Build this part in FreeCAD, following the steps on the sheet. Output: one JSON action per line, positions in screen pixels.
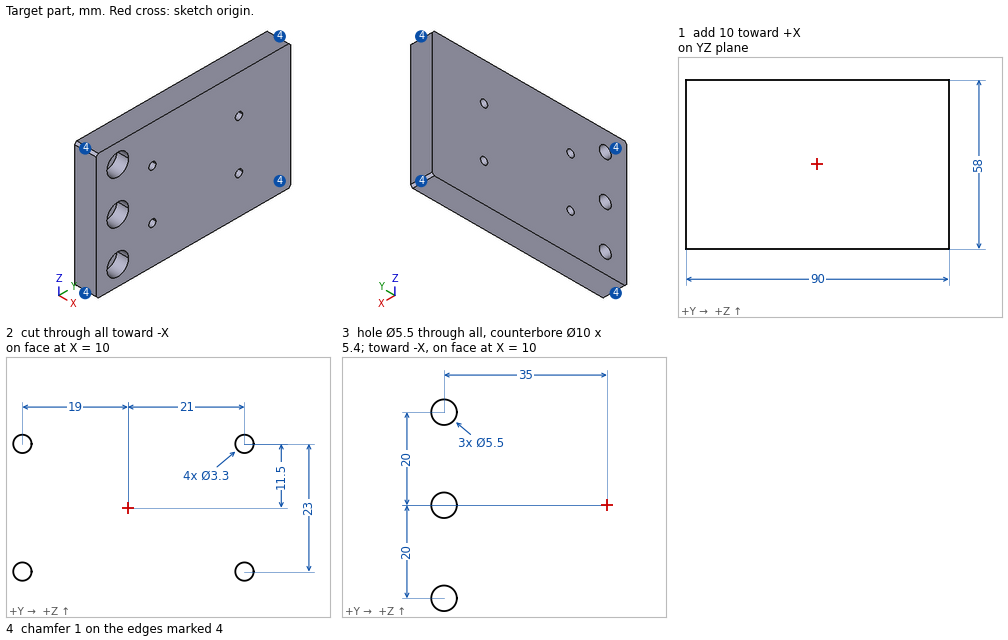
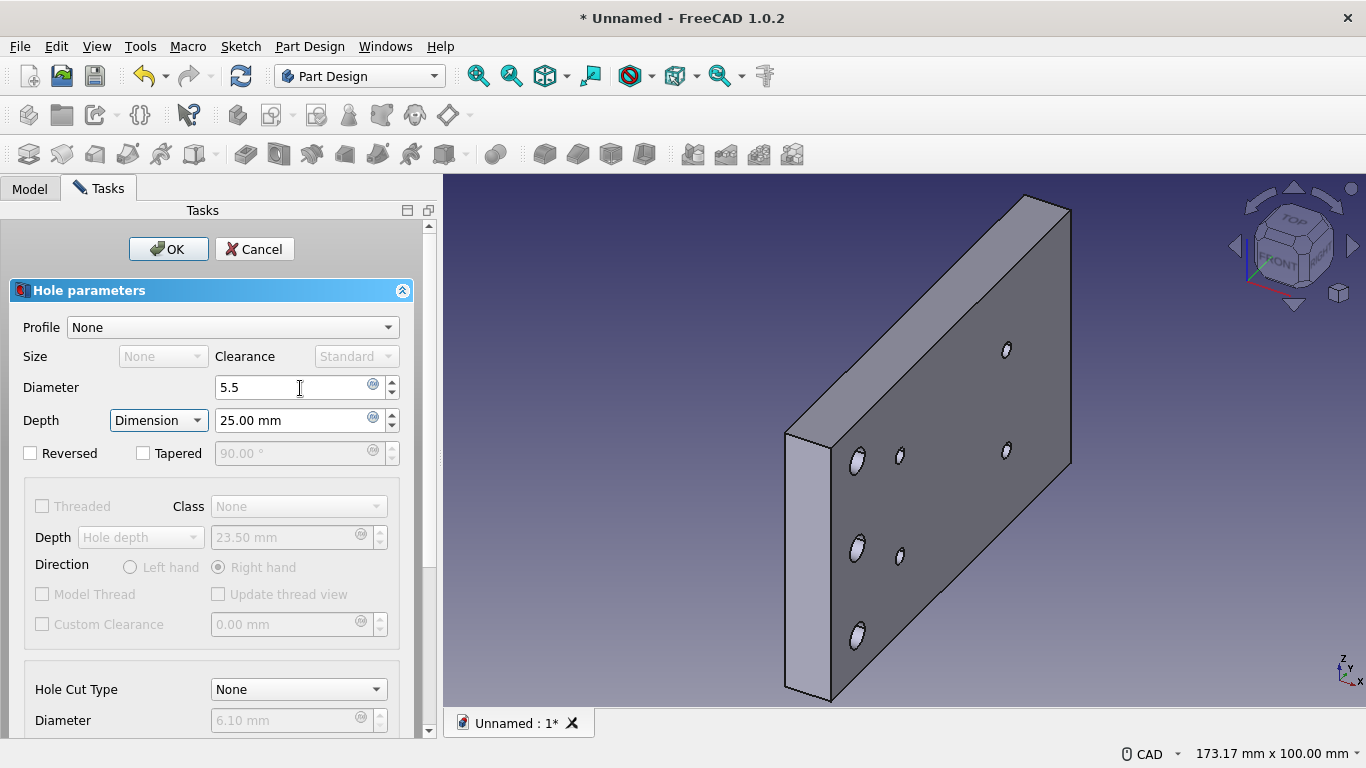
{"action": "left_click", "coordinate": [160, 420]}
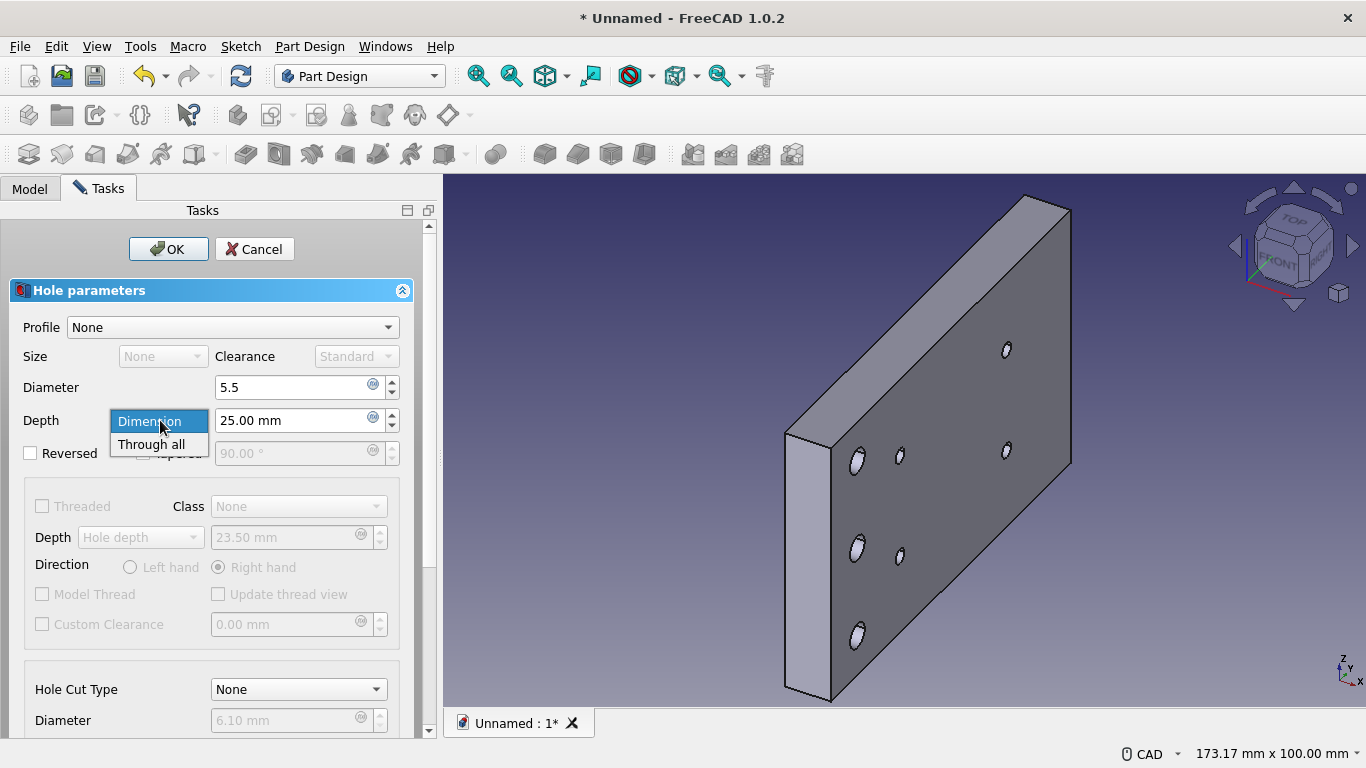
{"action": "left_click", "coordinate": [158, 444]}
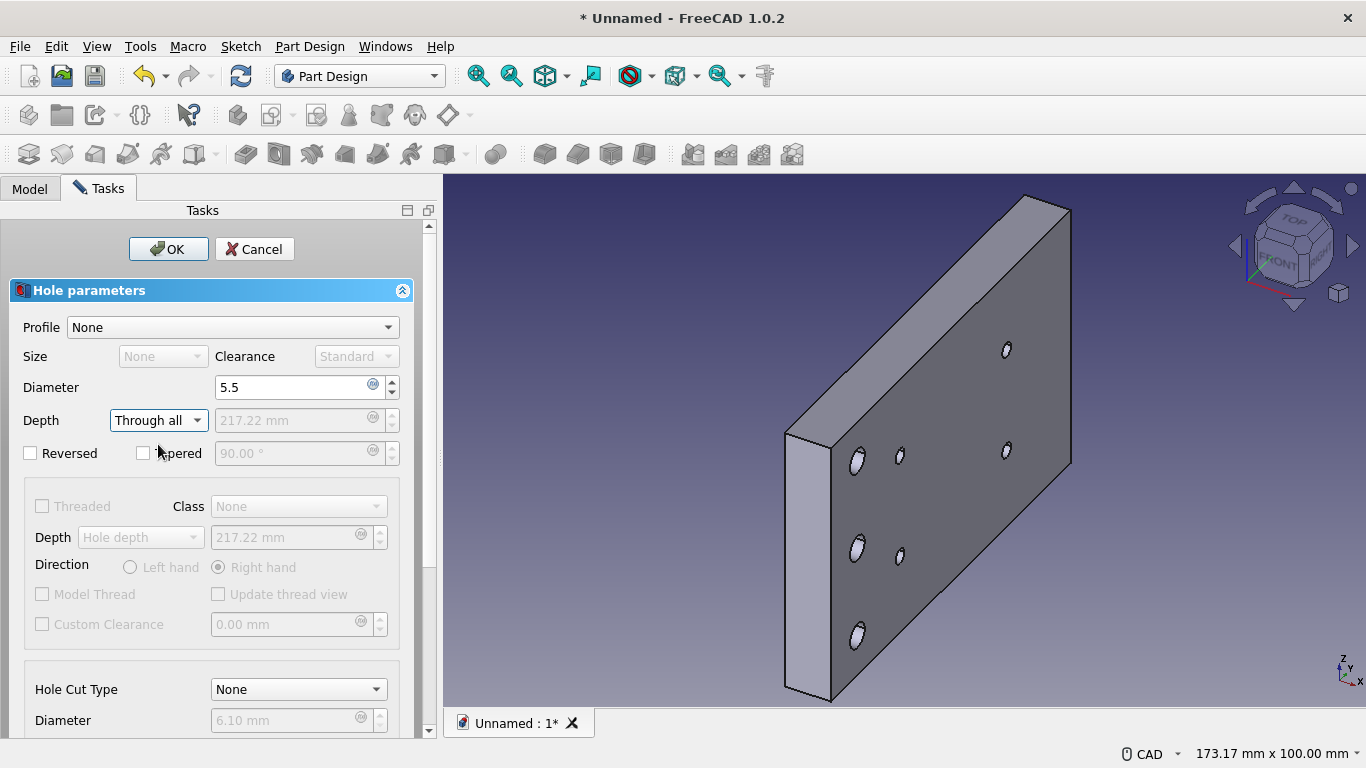
{"action": "left_click", "coordinate": [300, 690]}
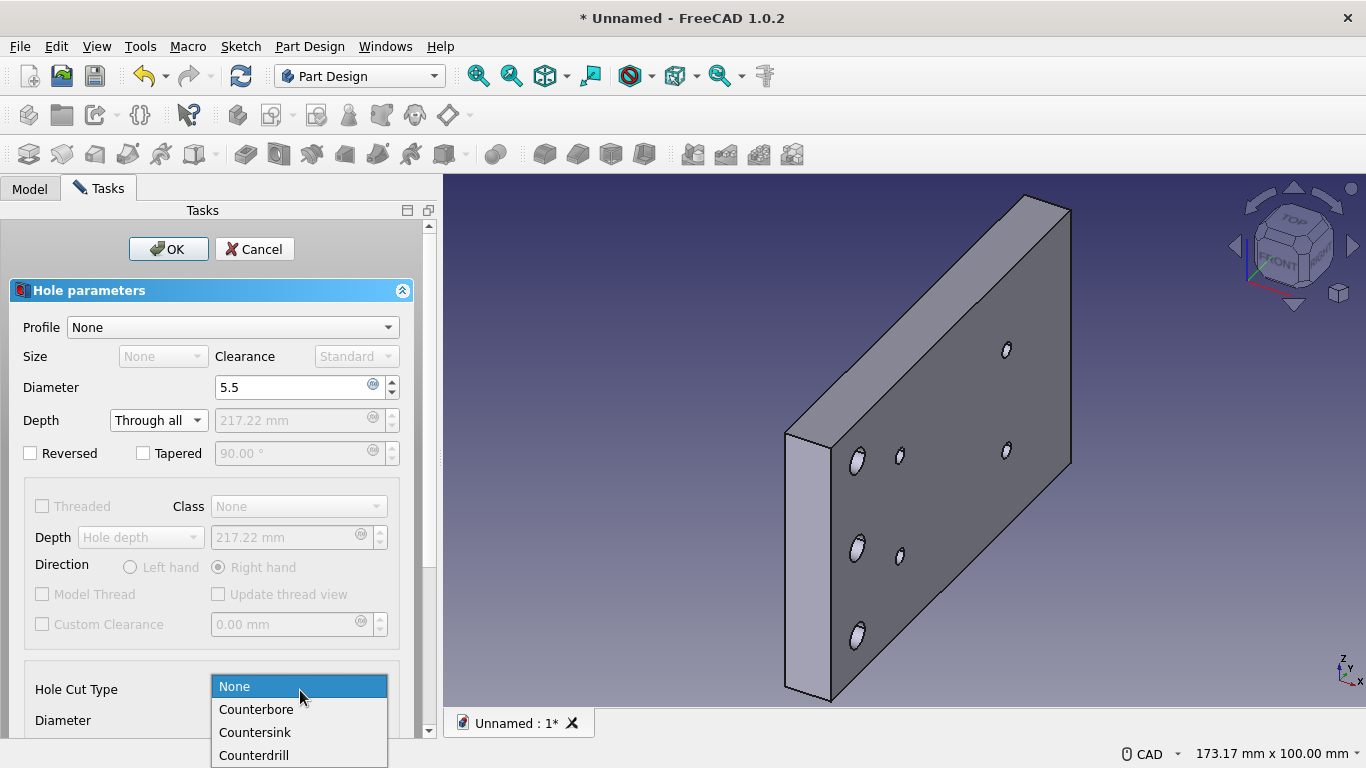
{"action": "left_click", "coordinate": [298, 710]}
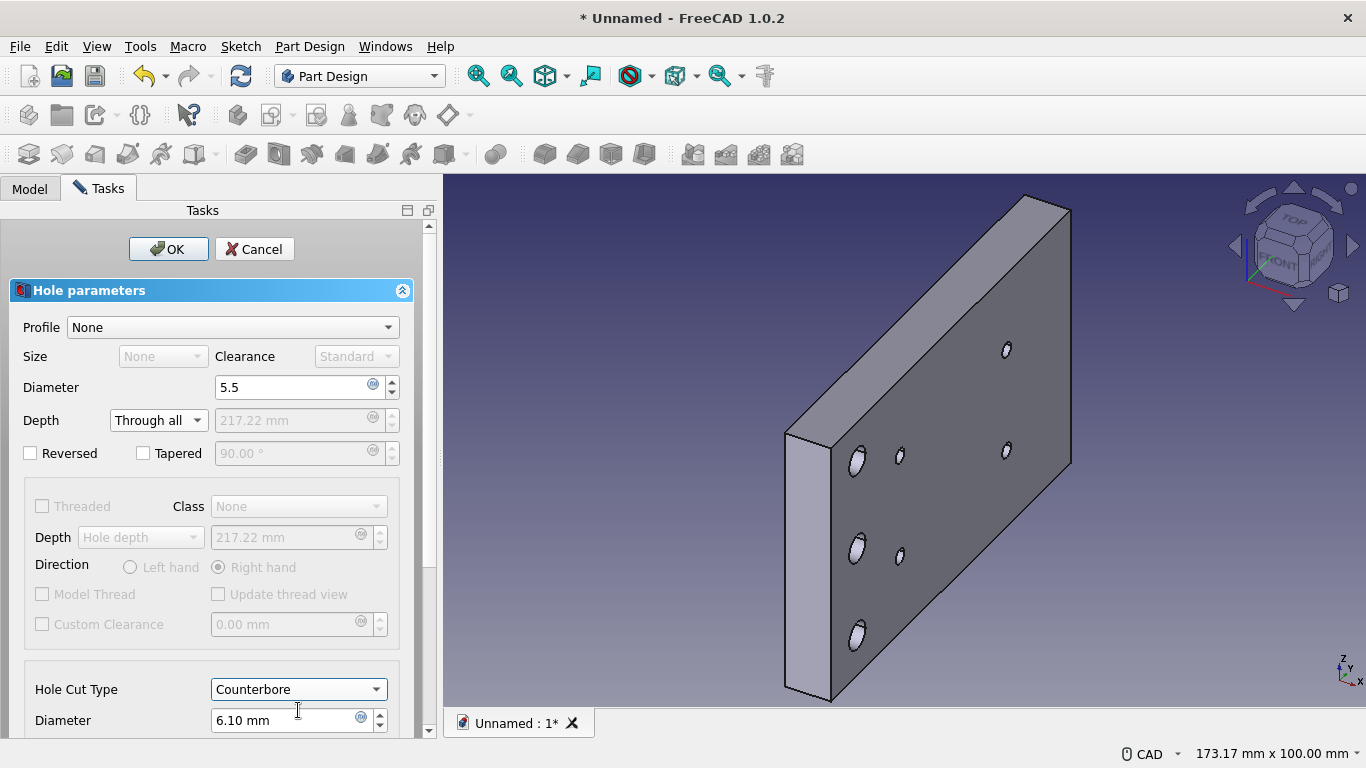
{"action": "triple_click", "coordinate": [292, 720]}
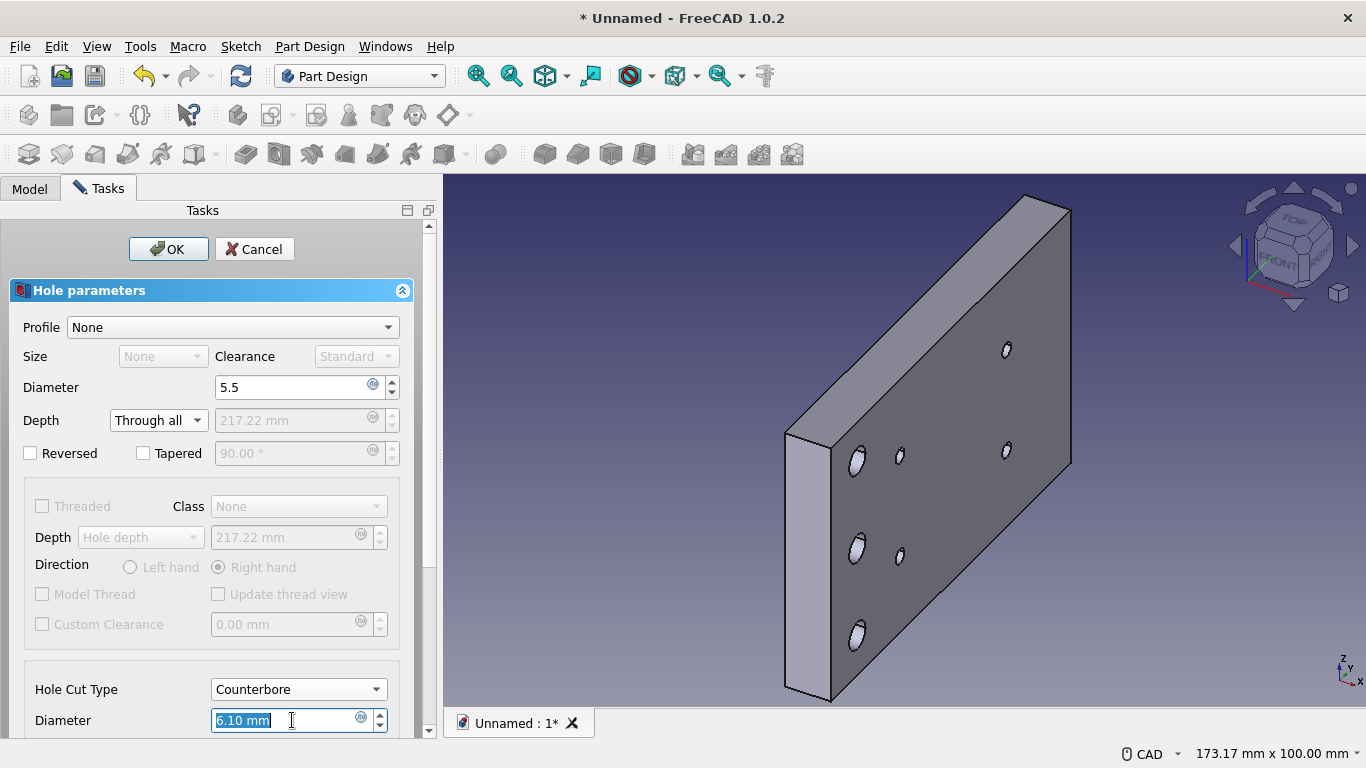
{"action": "type", "text": "10"}
{"action": "key", "text": "Tab"}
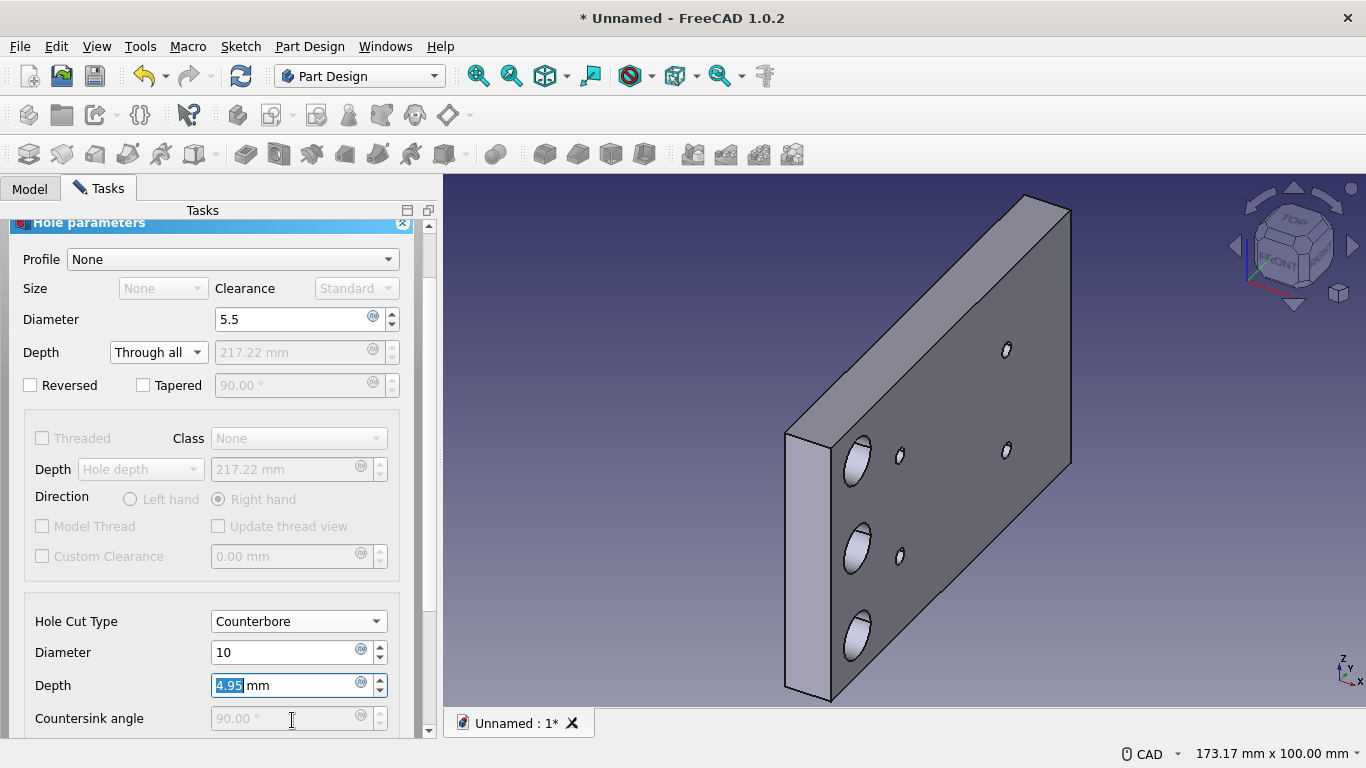
{"action": "type", "text": "5.4"}
{"action": "key", "text": "Tab"}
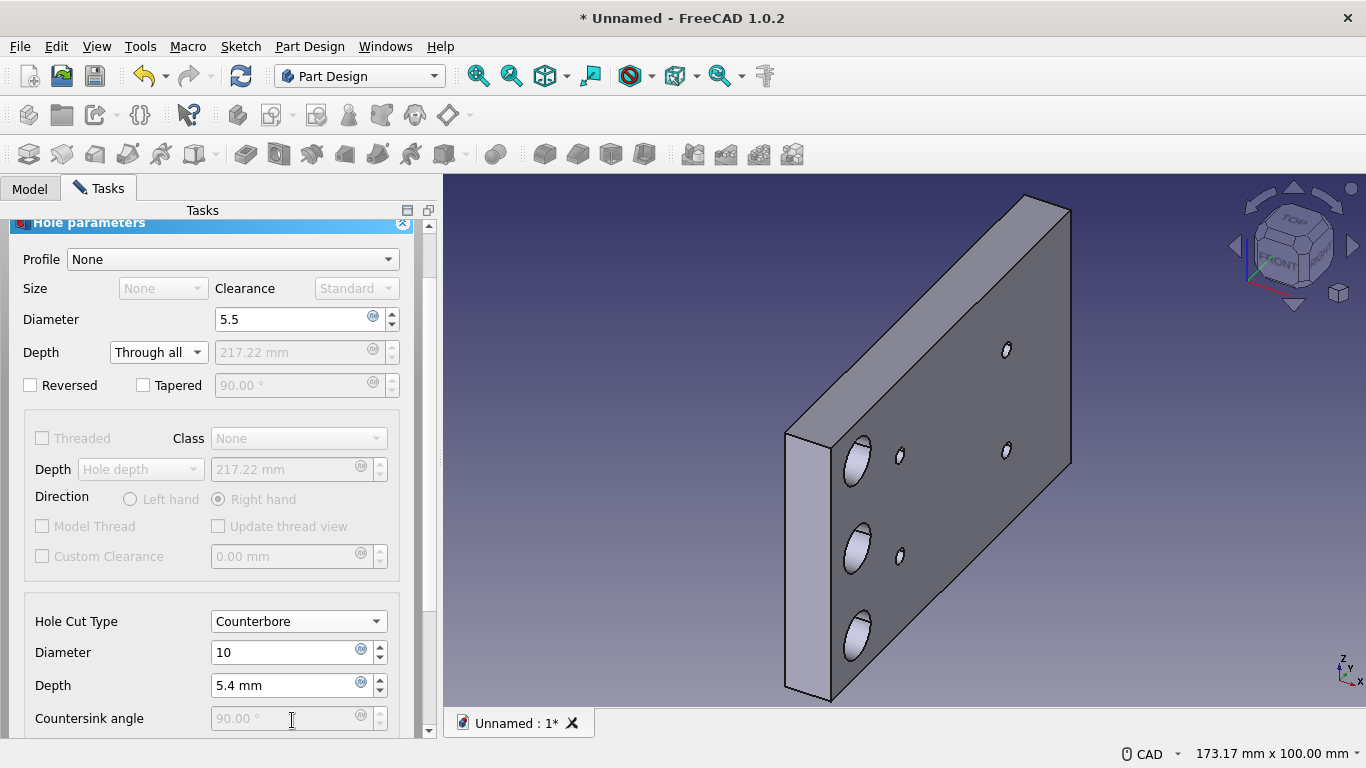
{"action": "scroll", "coordinate": [429, 479], "scroll_direction": "up", "scroll_amount": 2}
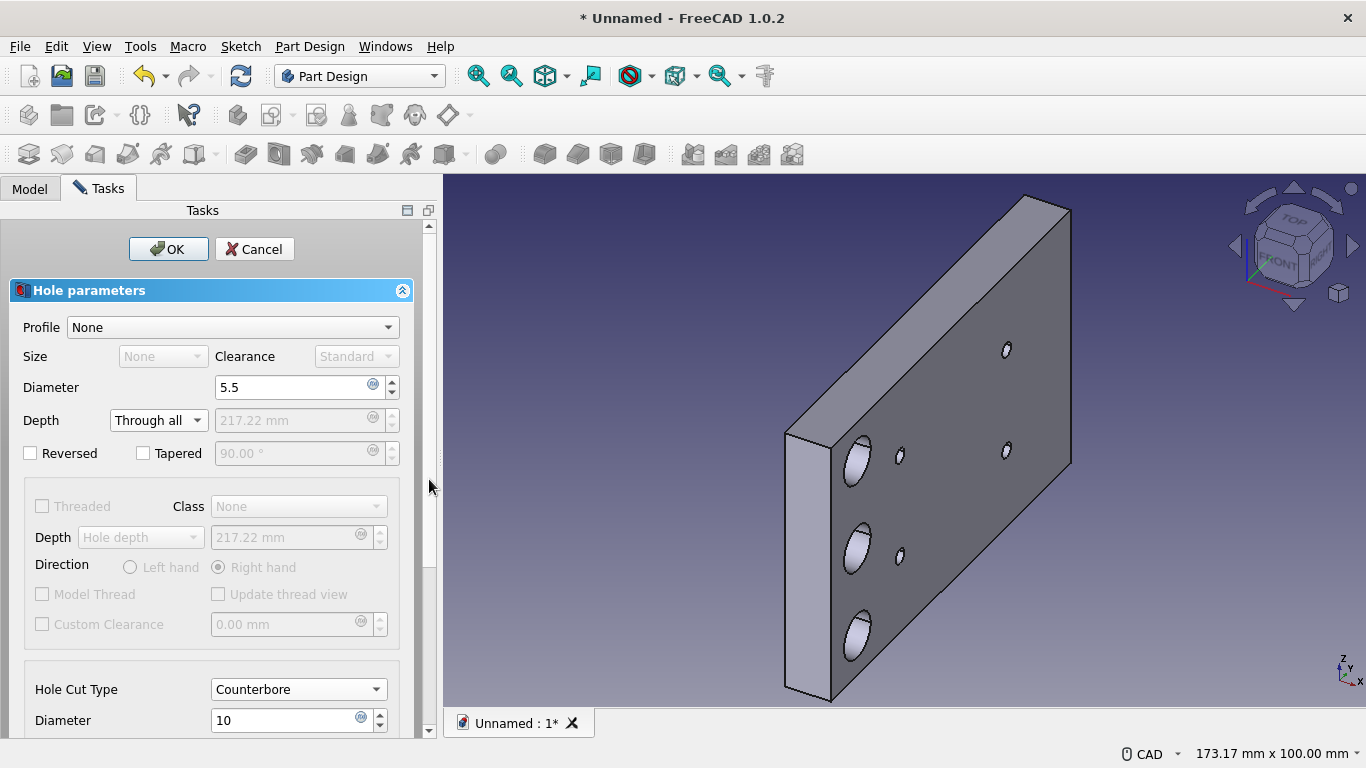
{"action": "left_click", "coordinate": [169, 249]}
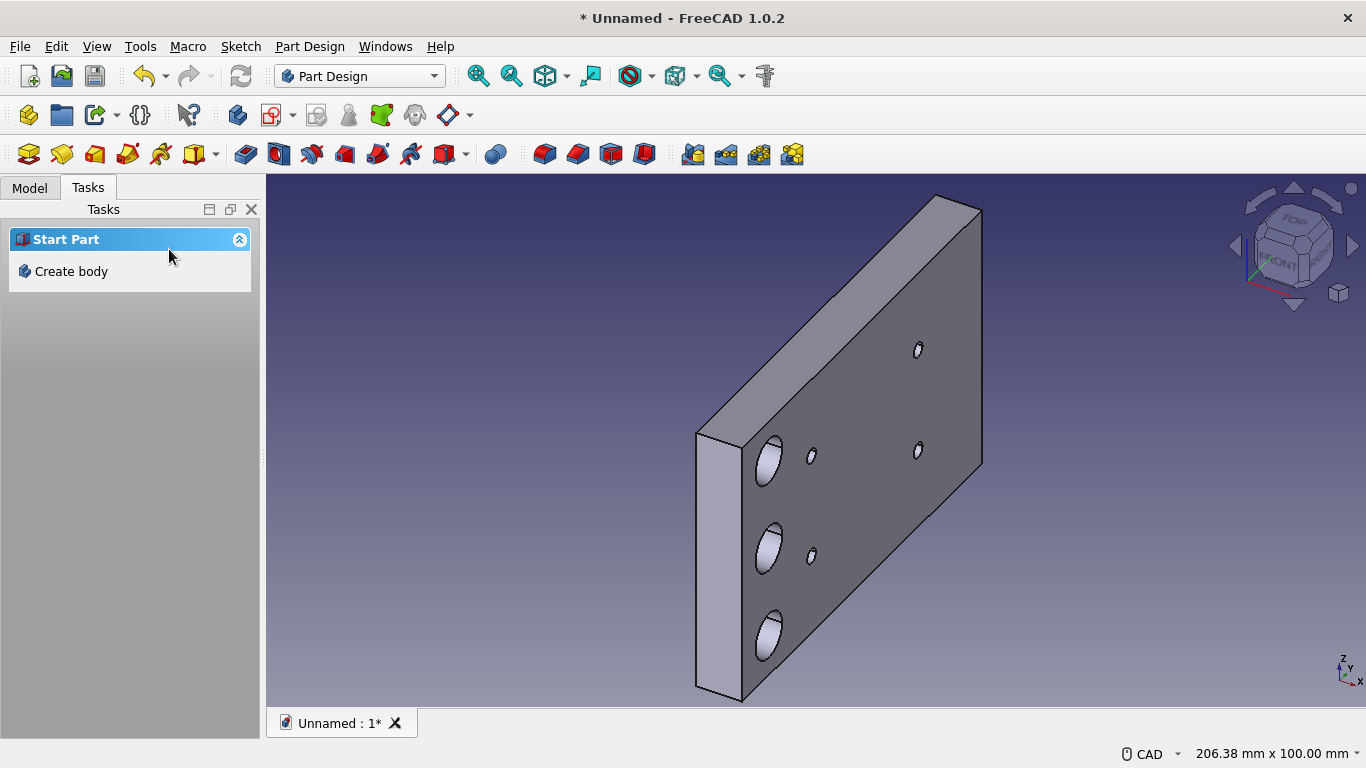
{"action": "left_click", "coordinate": [719, 440]}